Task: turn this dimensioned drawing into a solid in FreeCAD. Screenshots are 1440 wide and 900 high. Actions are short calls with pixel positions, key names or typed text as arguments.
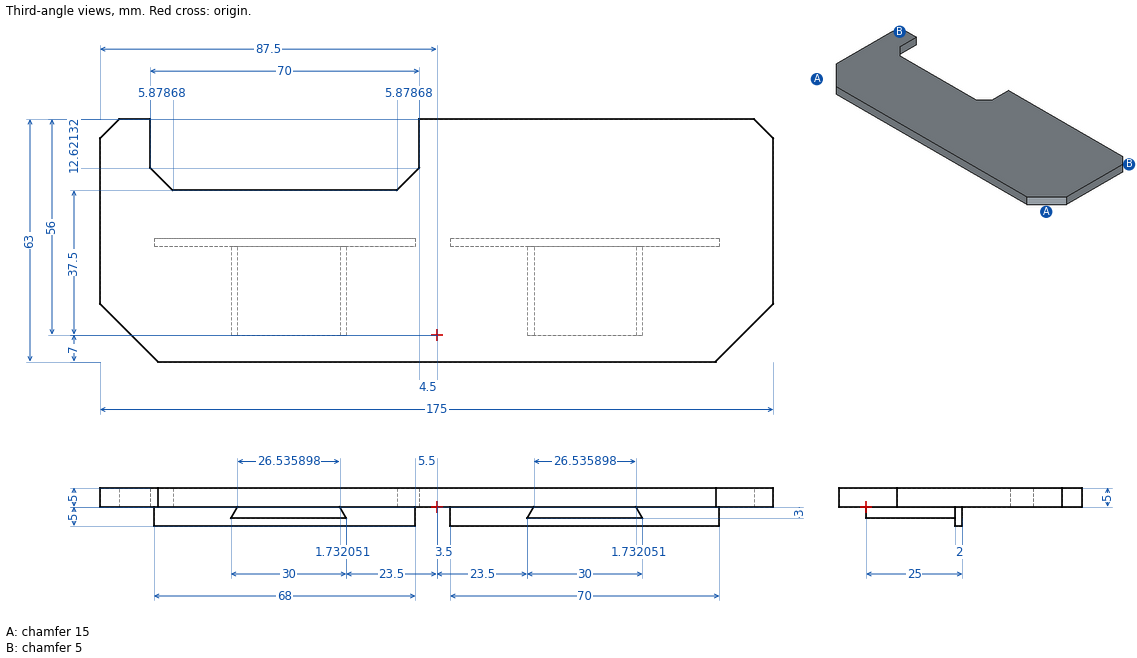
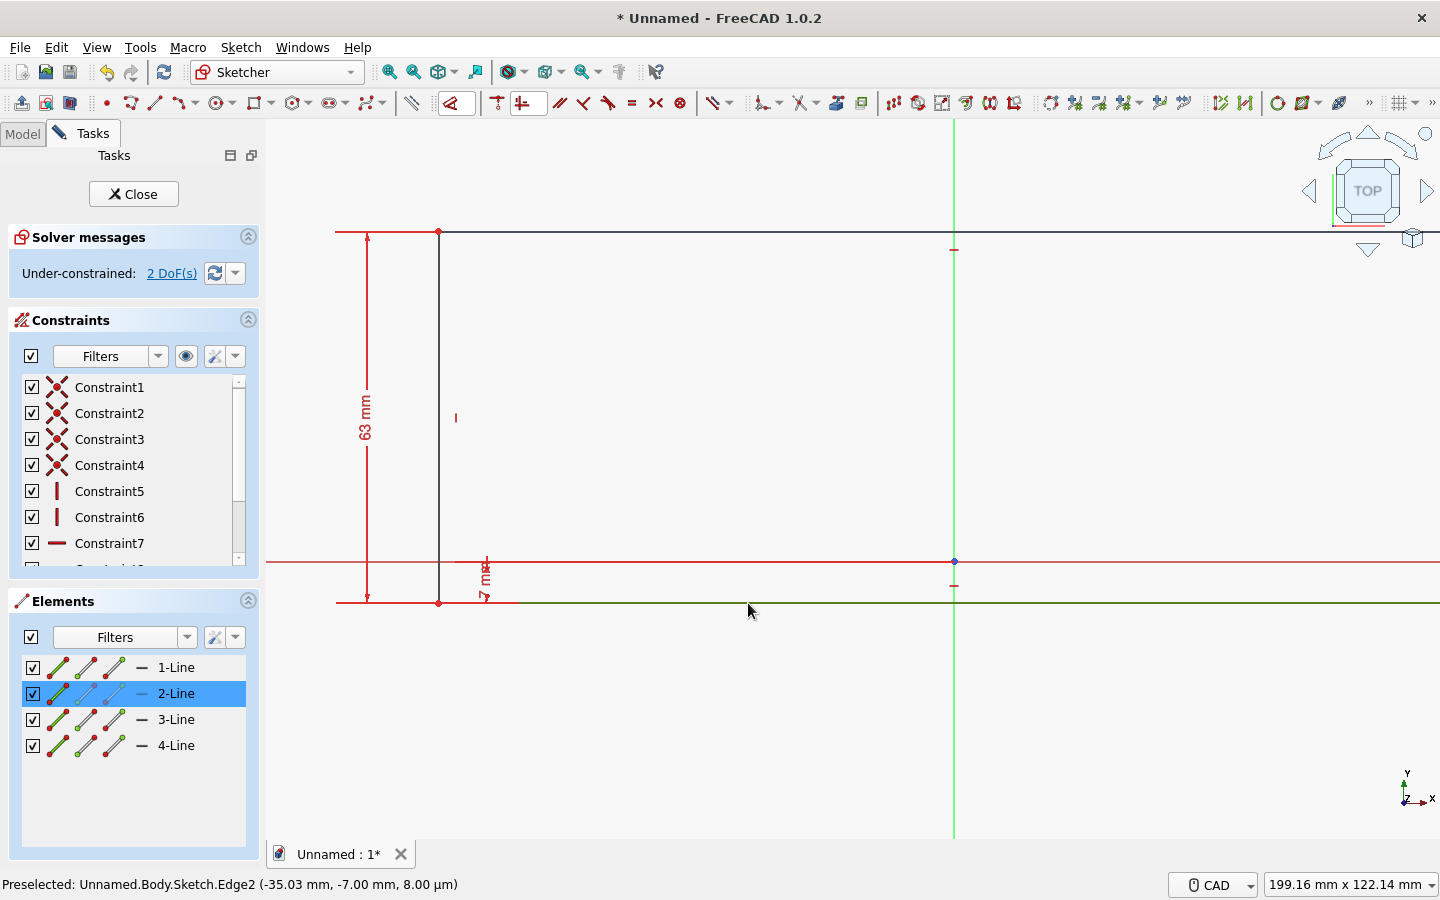
key(l)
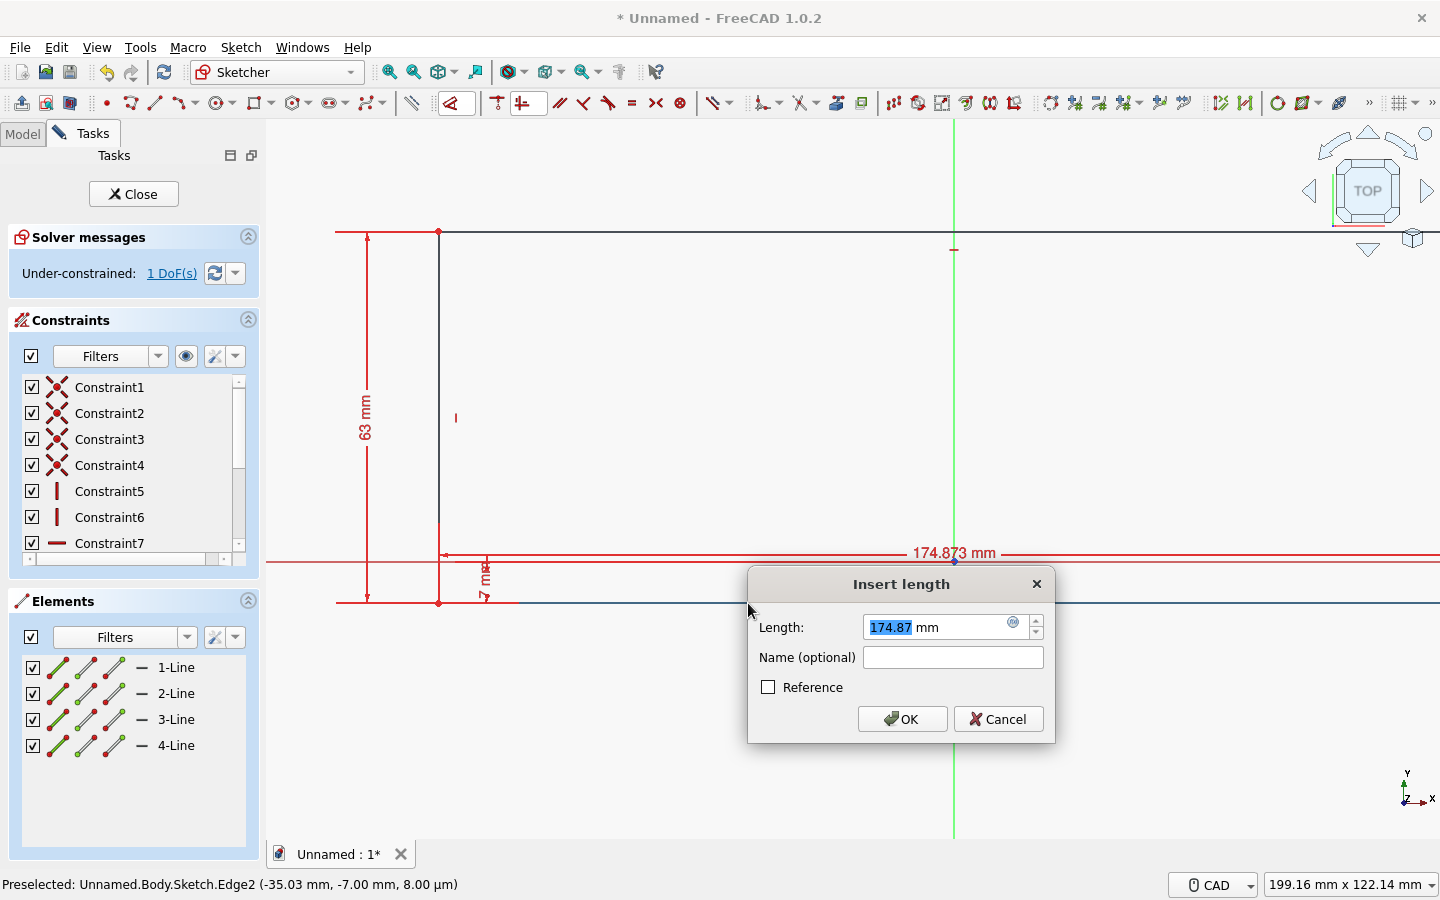
text(175)
key(Return)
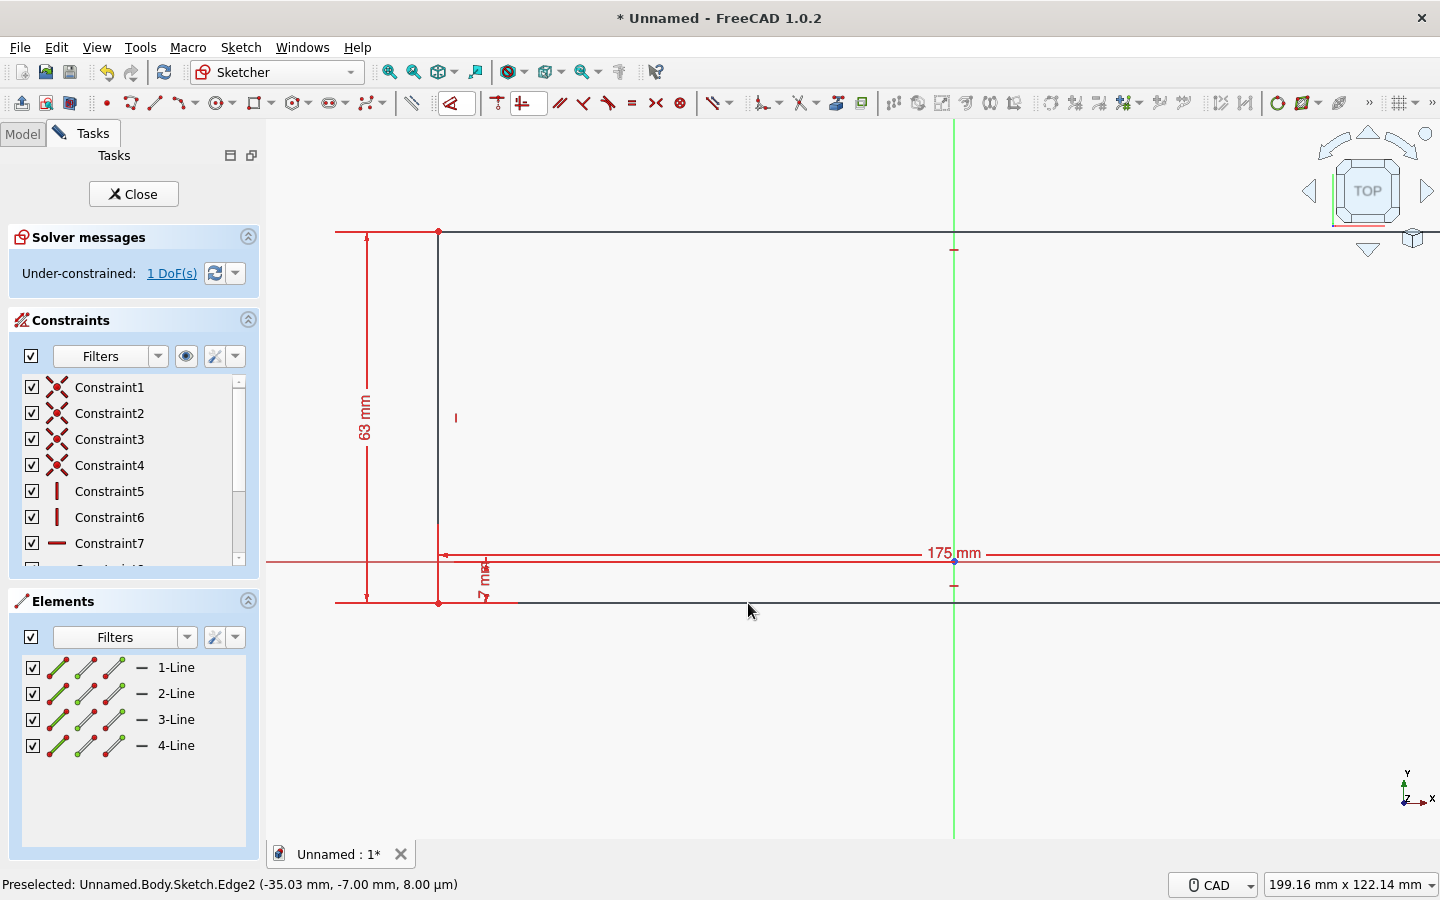
click(438, 232)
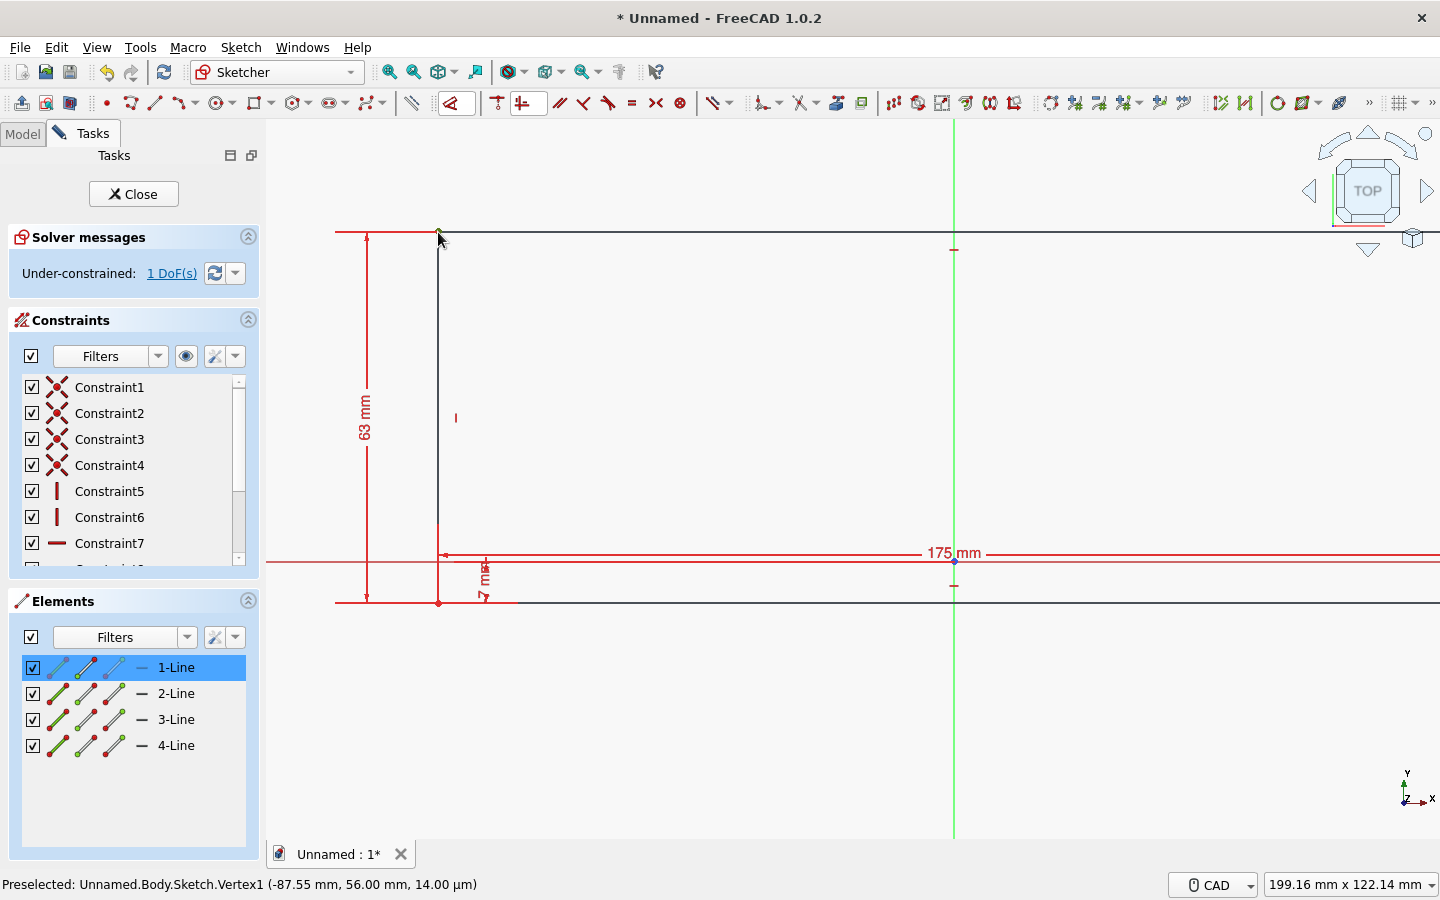
click(470, 104)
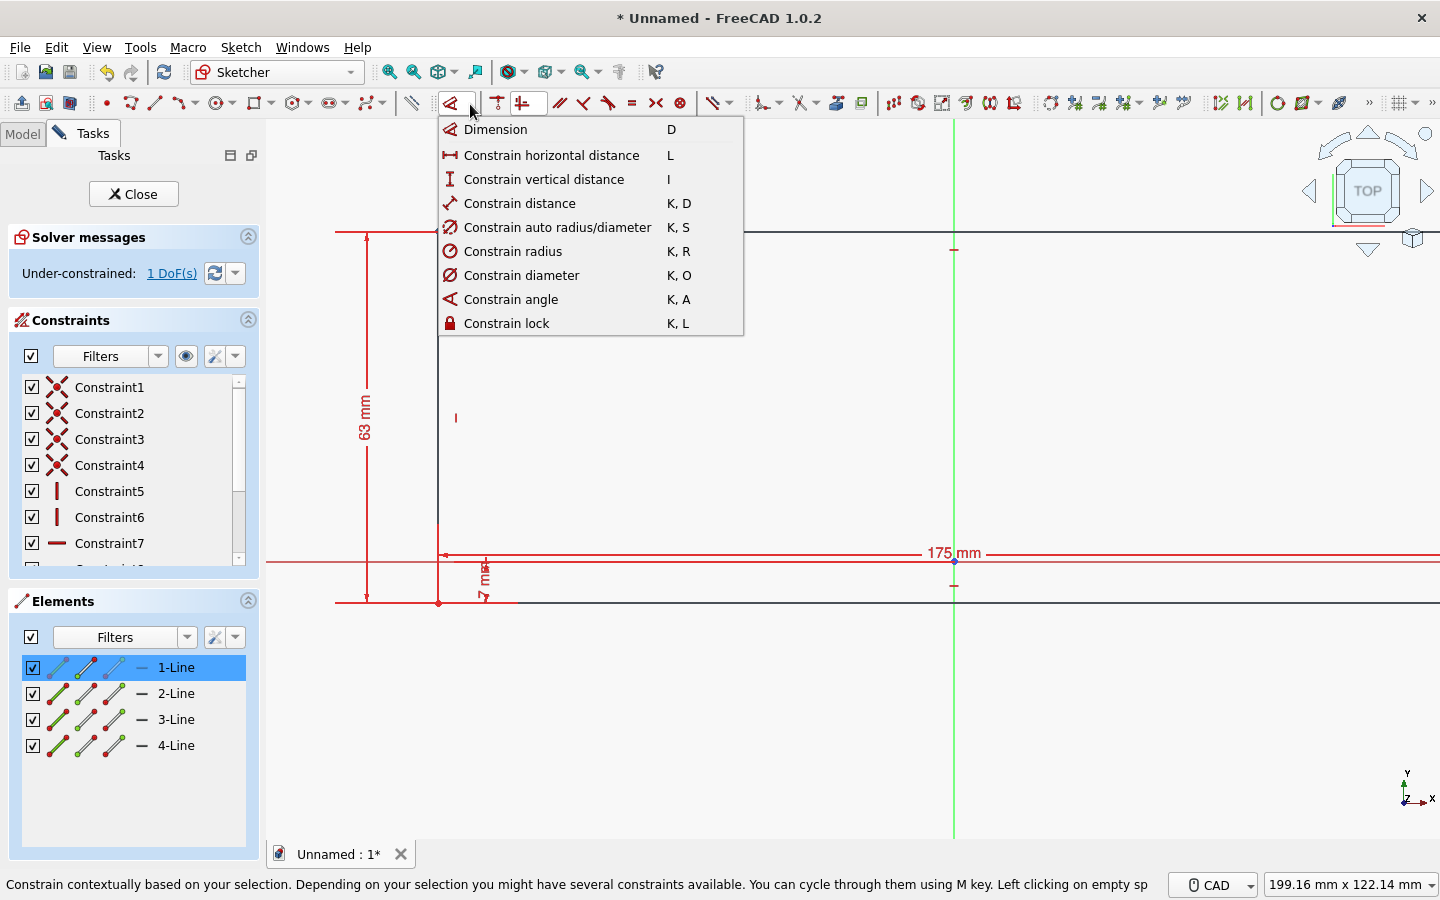
click(591, 155)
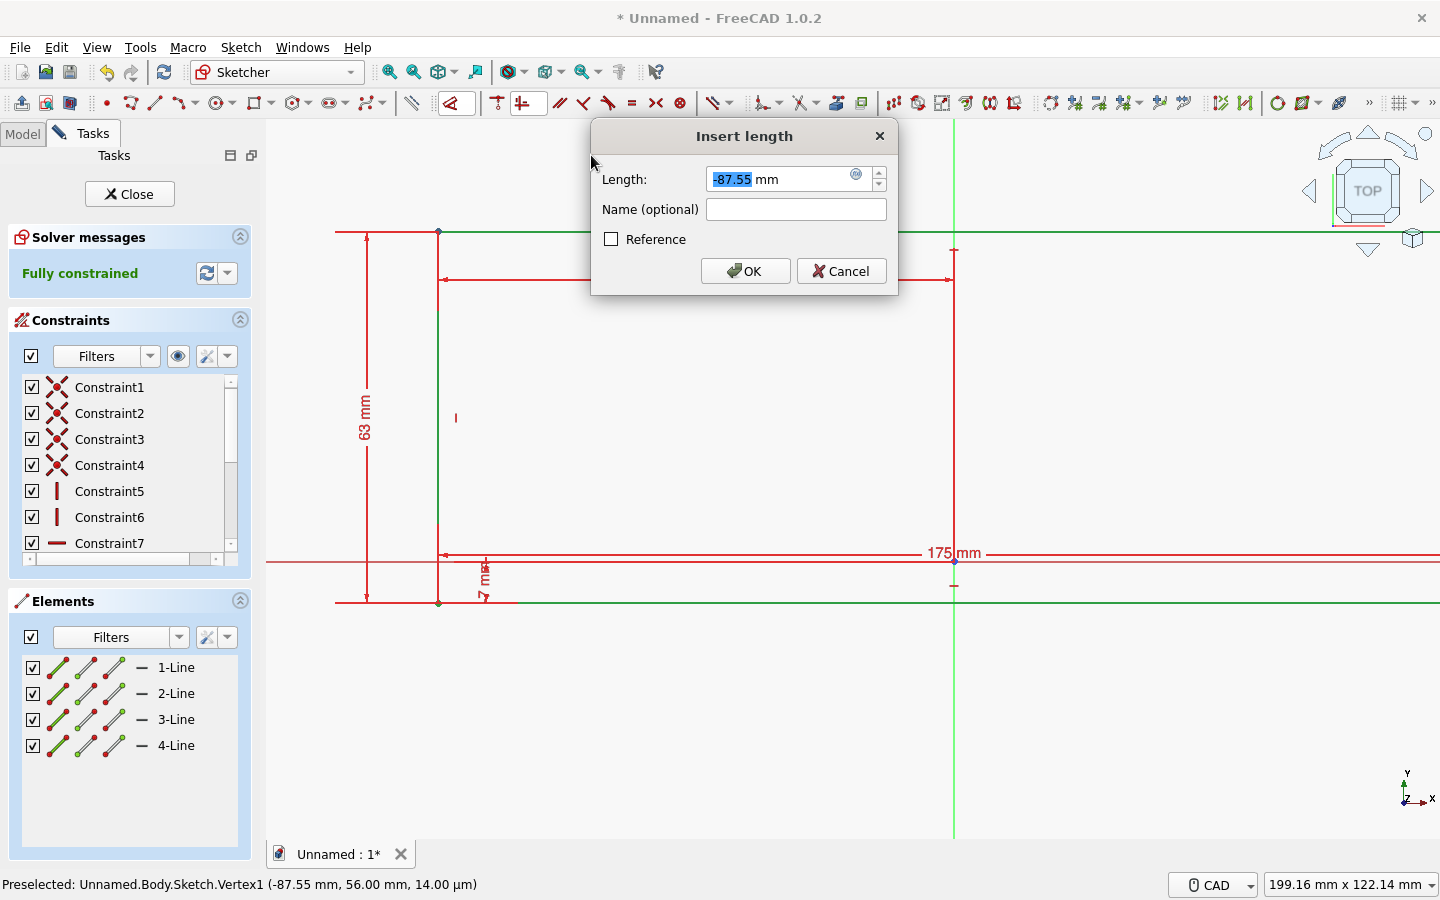
text(-87.5)
key(Return)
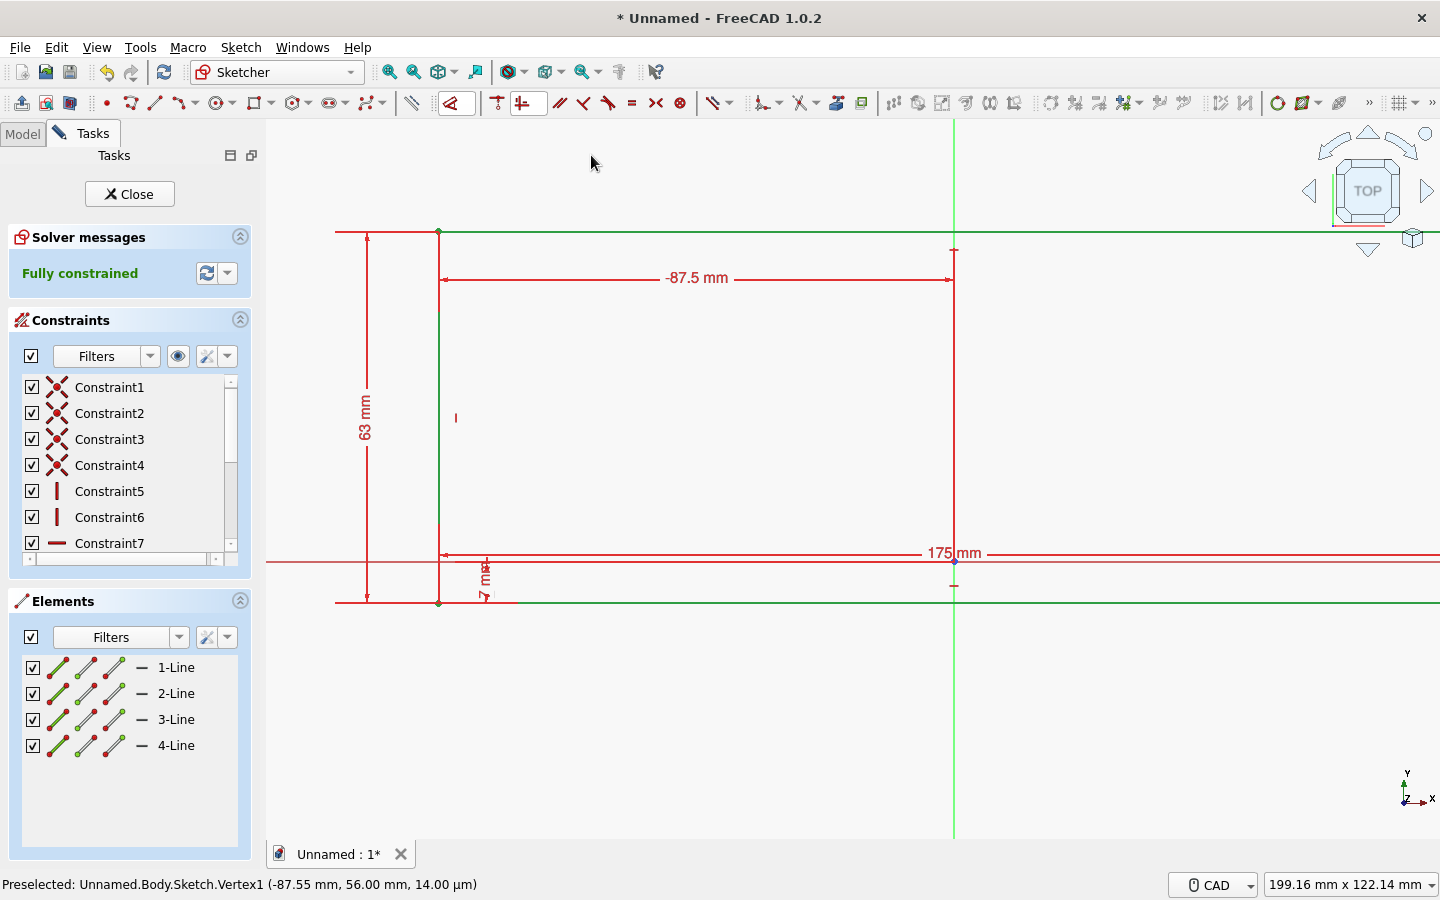
click(130, 194)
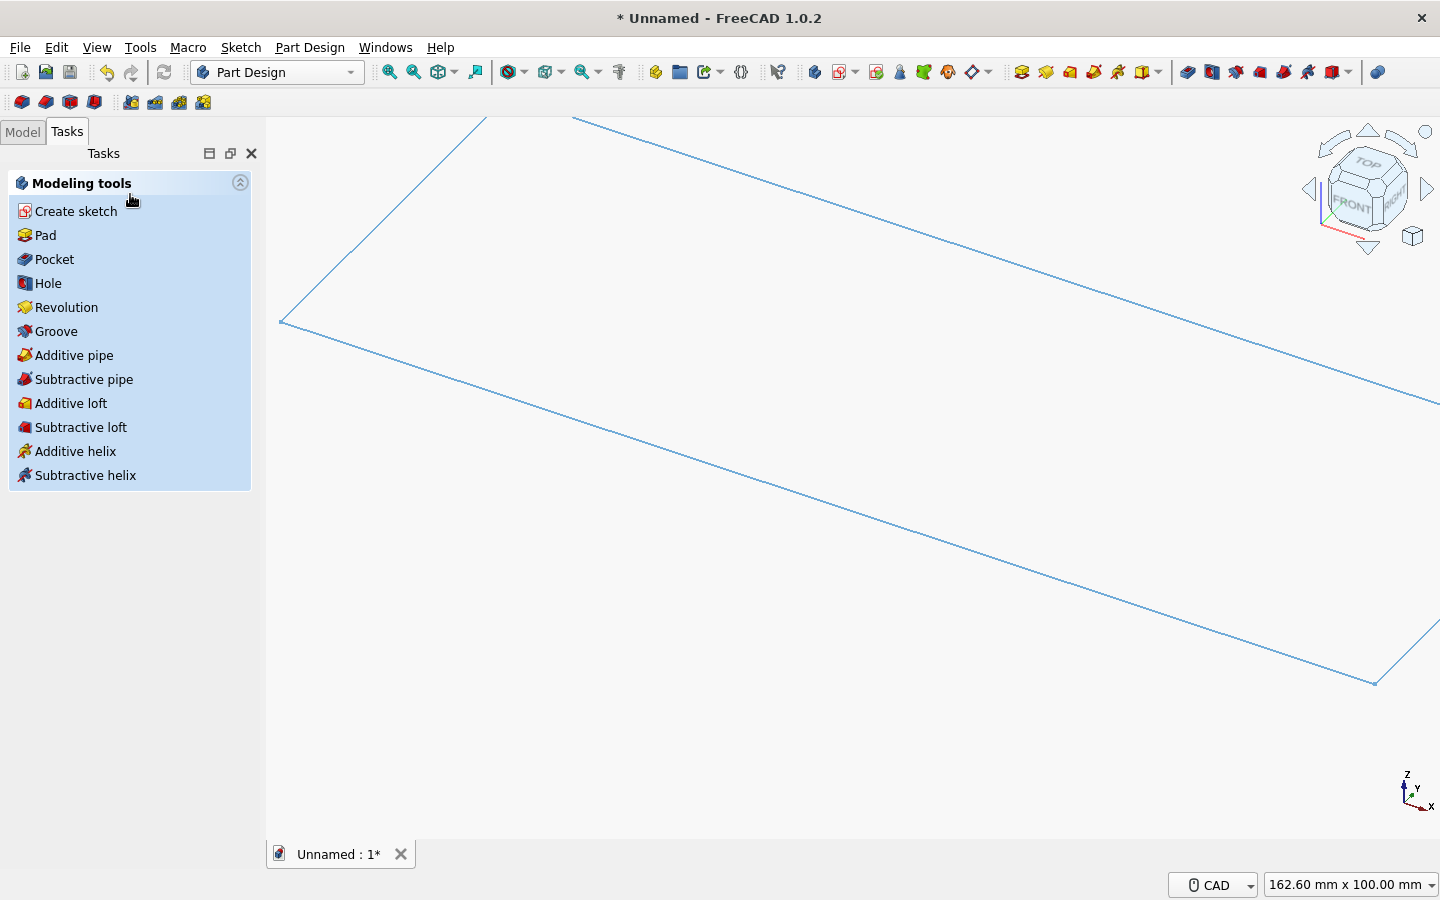
click(1022, 72)